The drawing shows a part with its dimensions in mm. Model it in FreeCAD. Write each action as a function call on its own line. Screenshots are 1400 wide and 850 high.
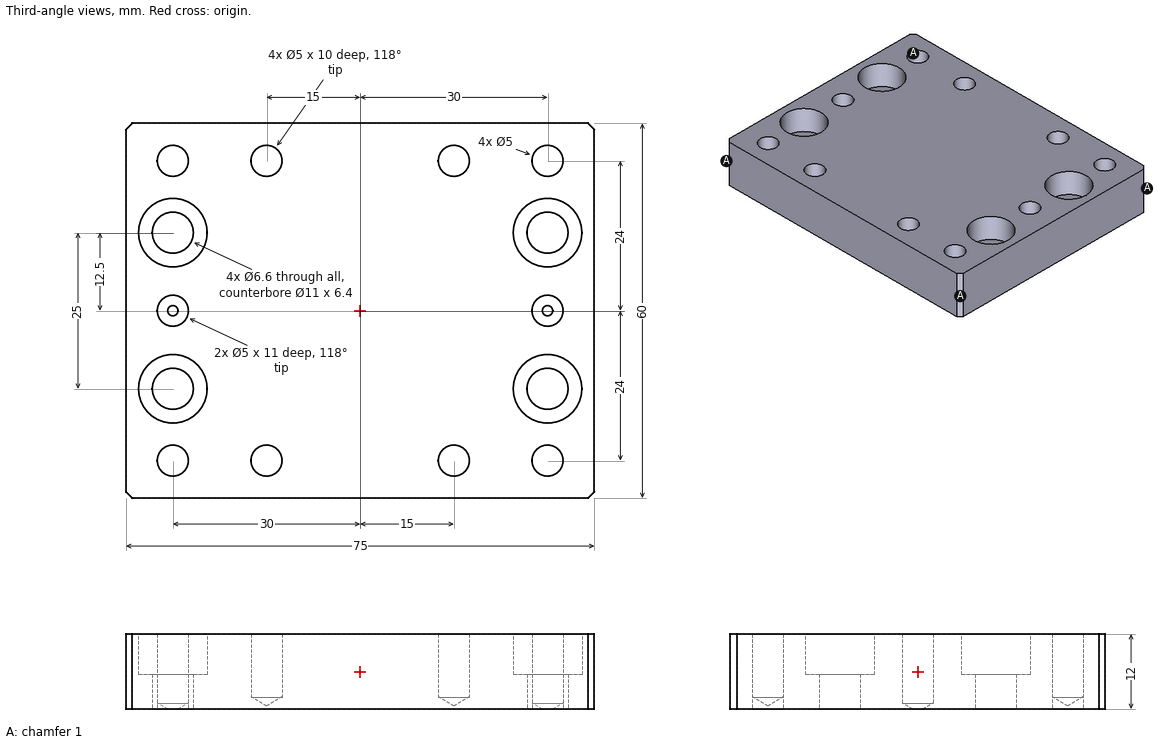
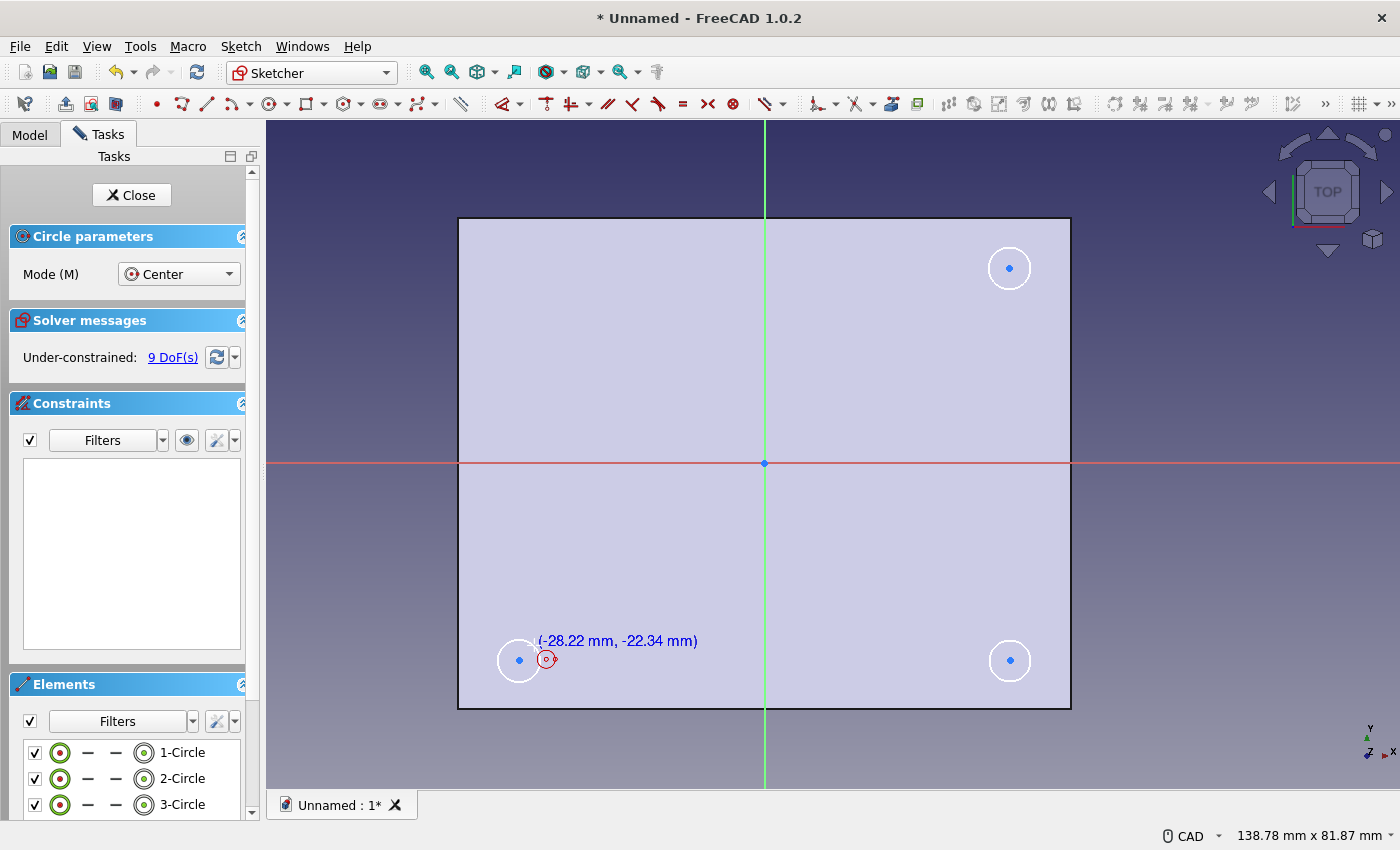
click(519, 267)
click(534, 253)
key(Escape)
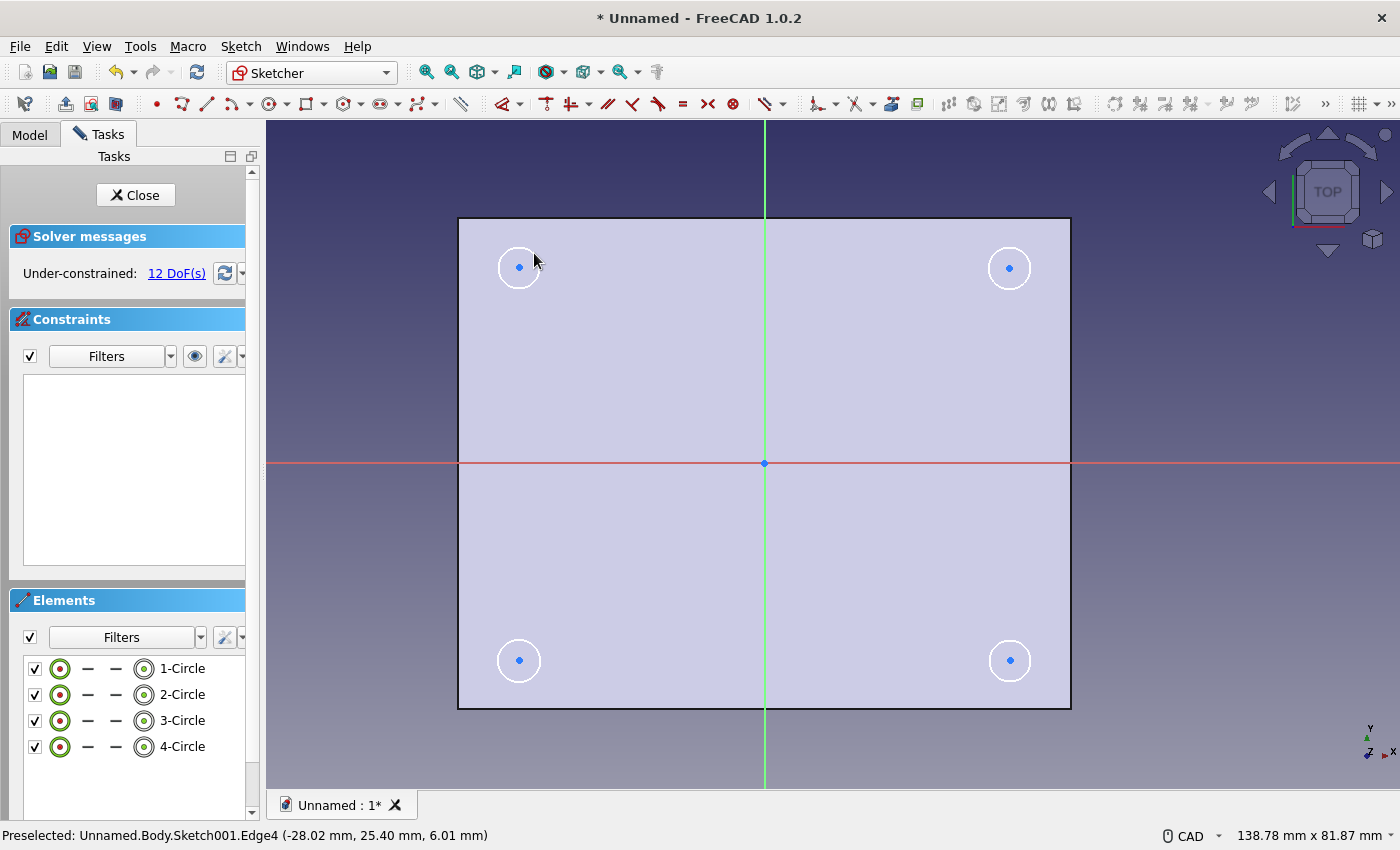
click(1024, 254)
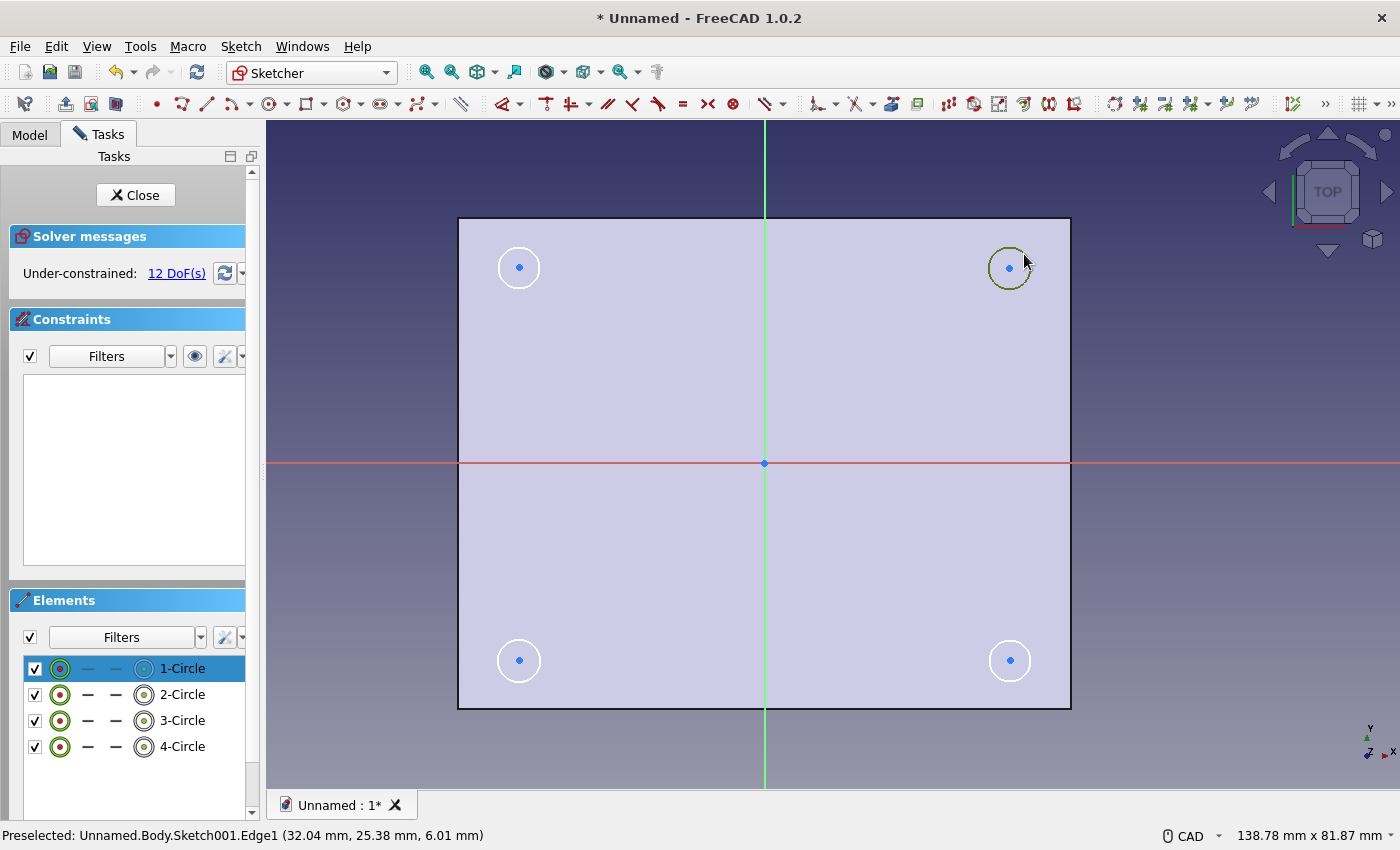
click(1024, 646)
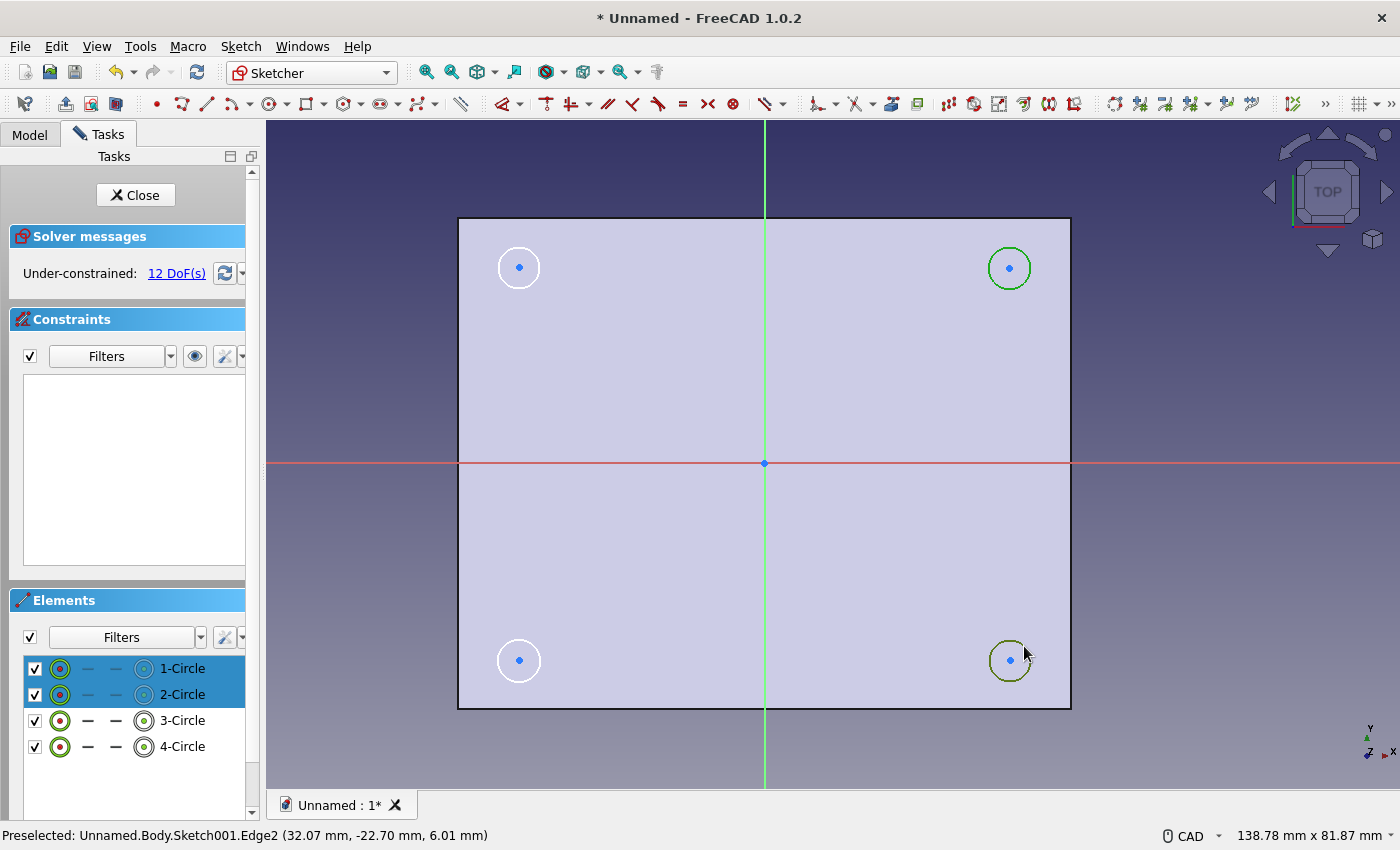
click(534, 646)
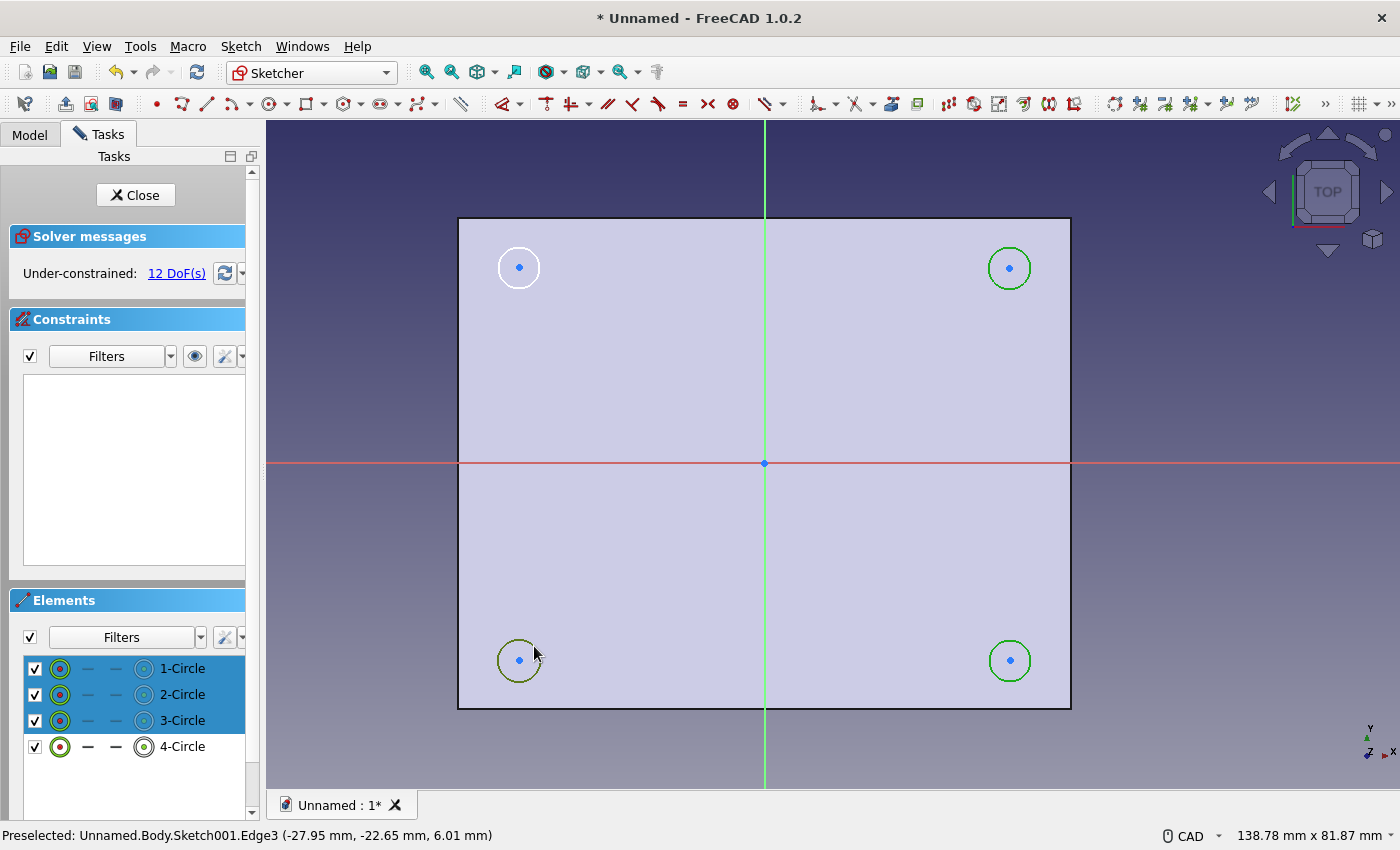
click(533, 253)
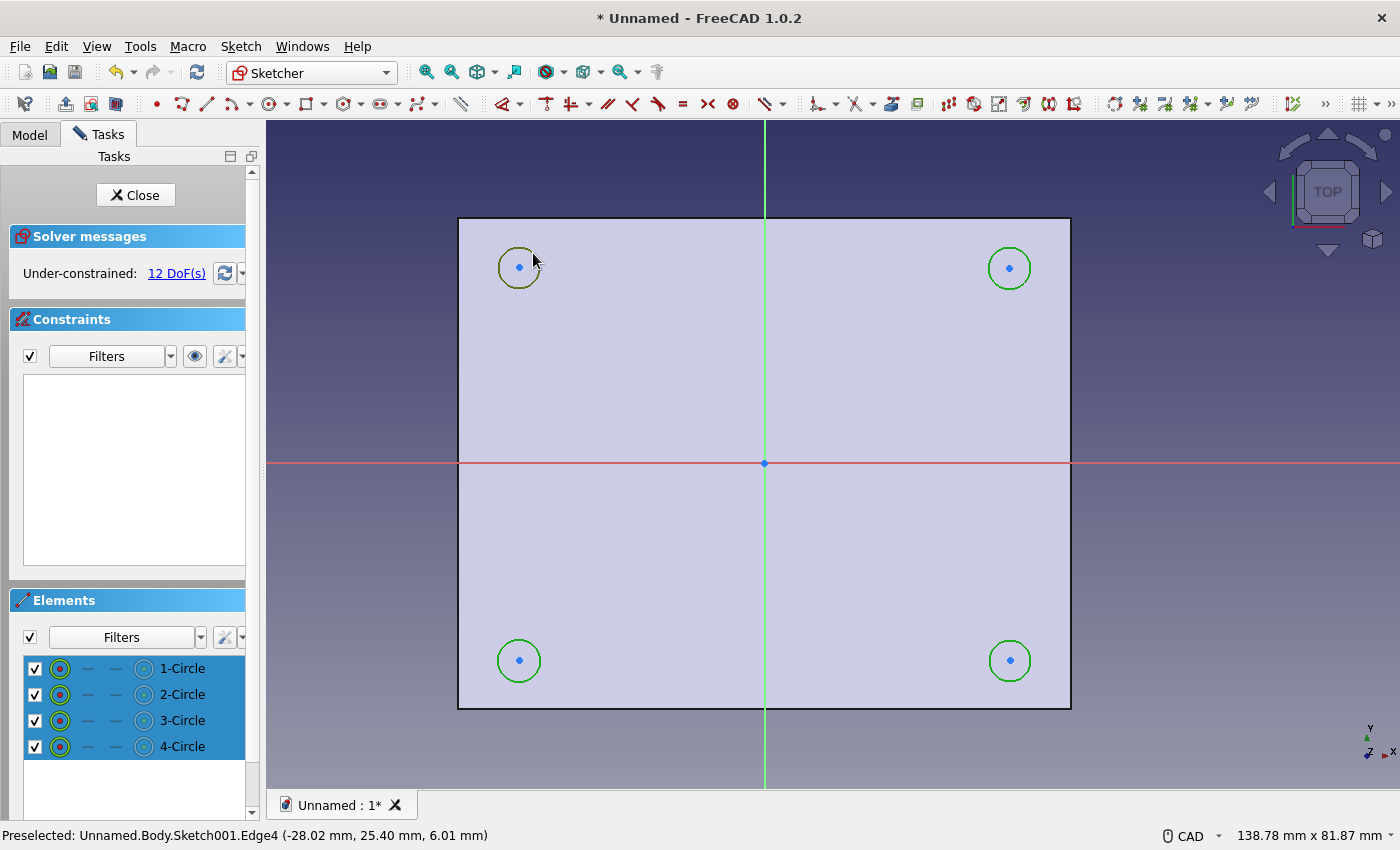
key(e)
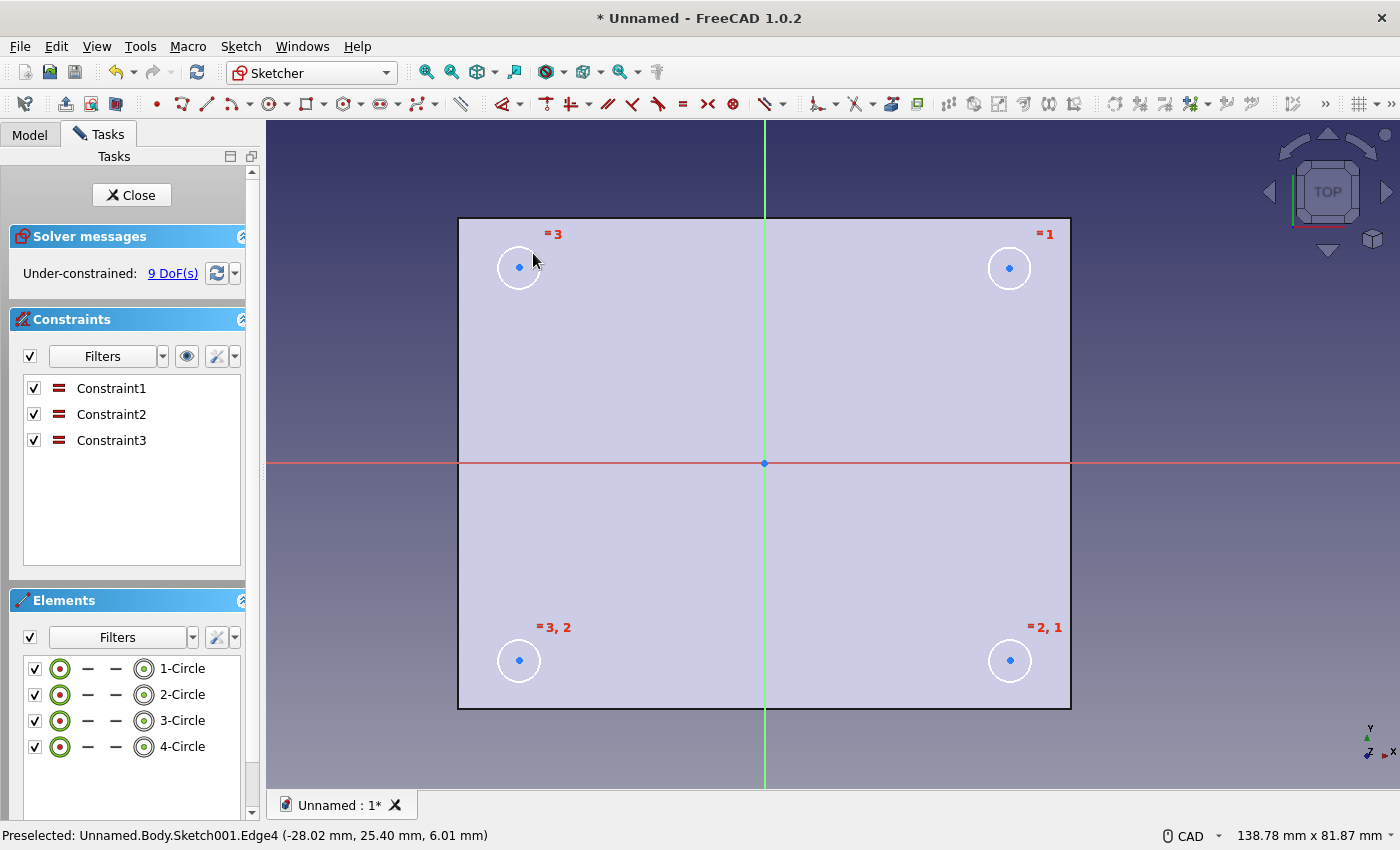
key(d)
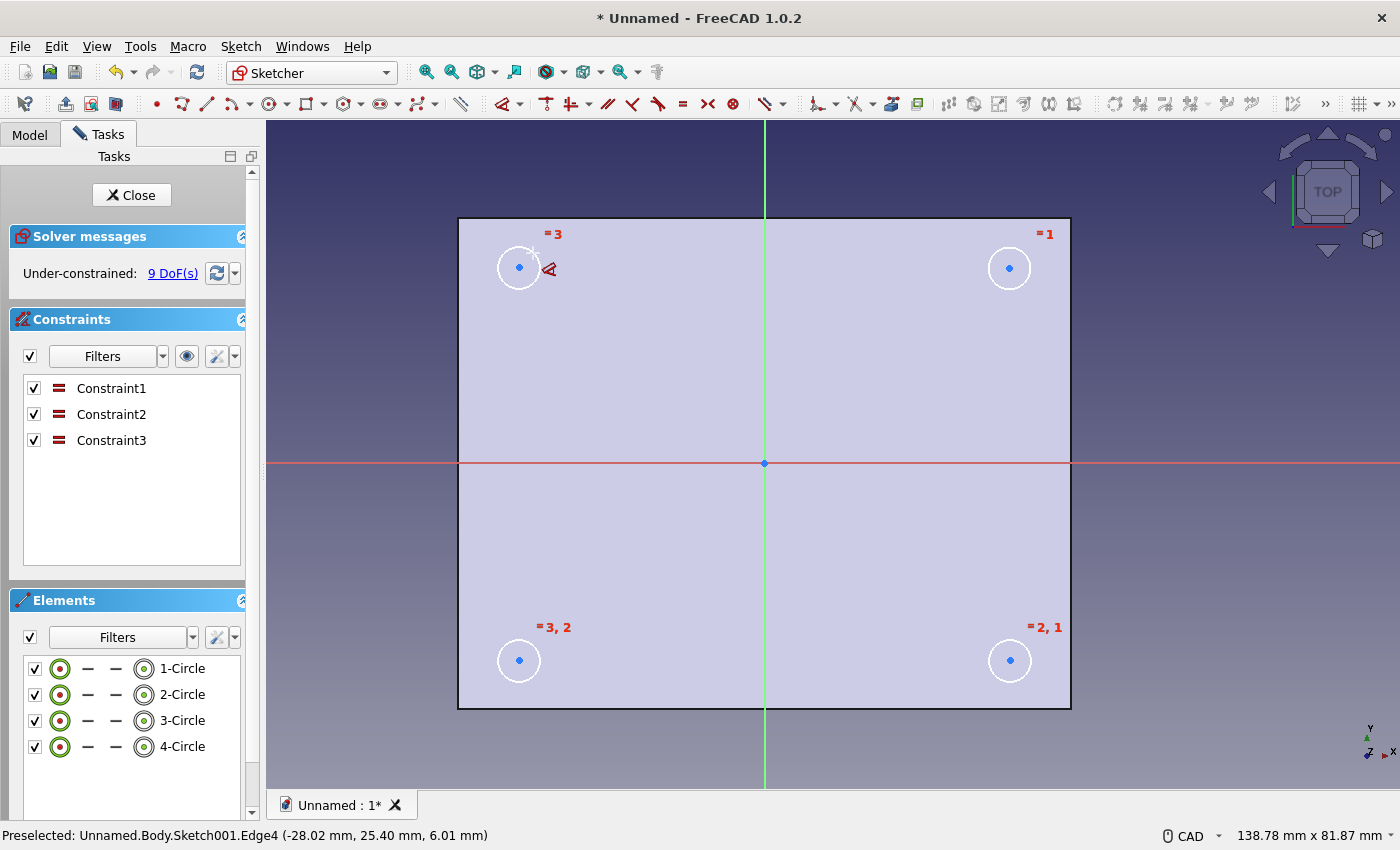
click(1024, 254)
click(1047, 231)